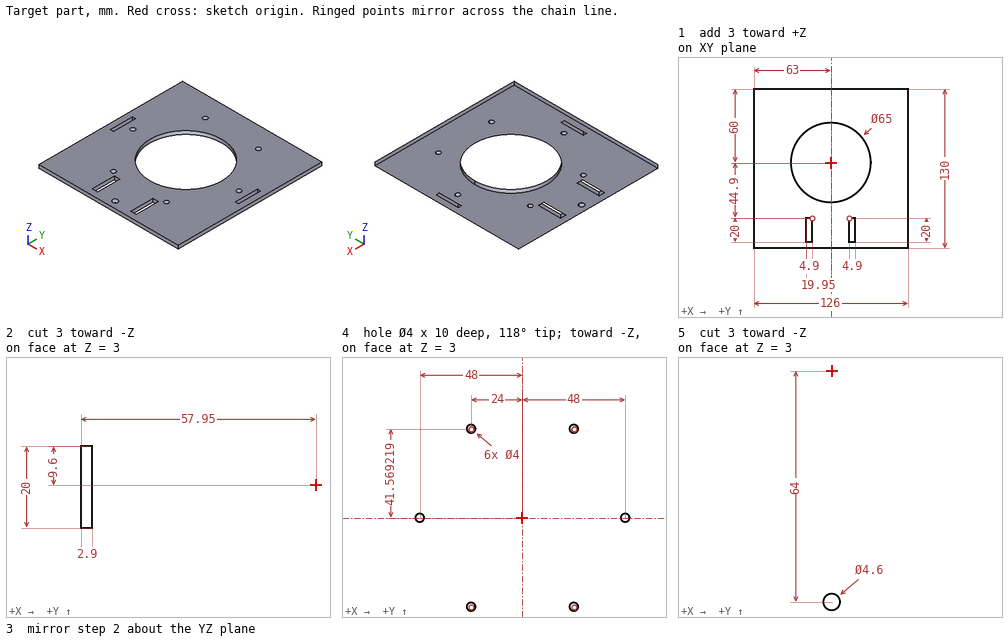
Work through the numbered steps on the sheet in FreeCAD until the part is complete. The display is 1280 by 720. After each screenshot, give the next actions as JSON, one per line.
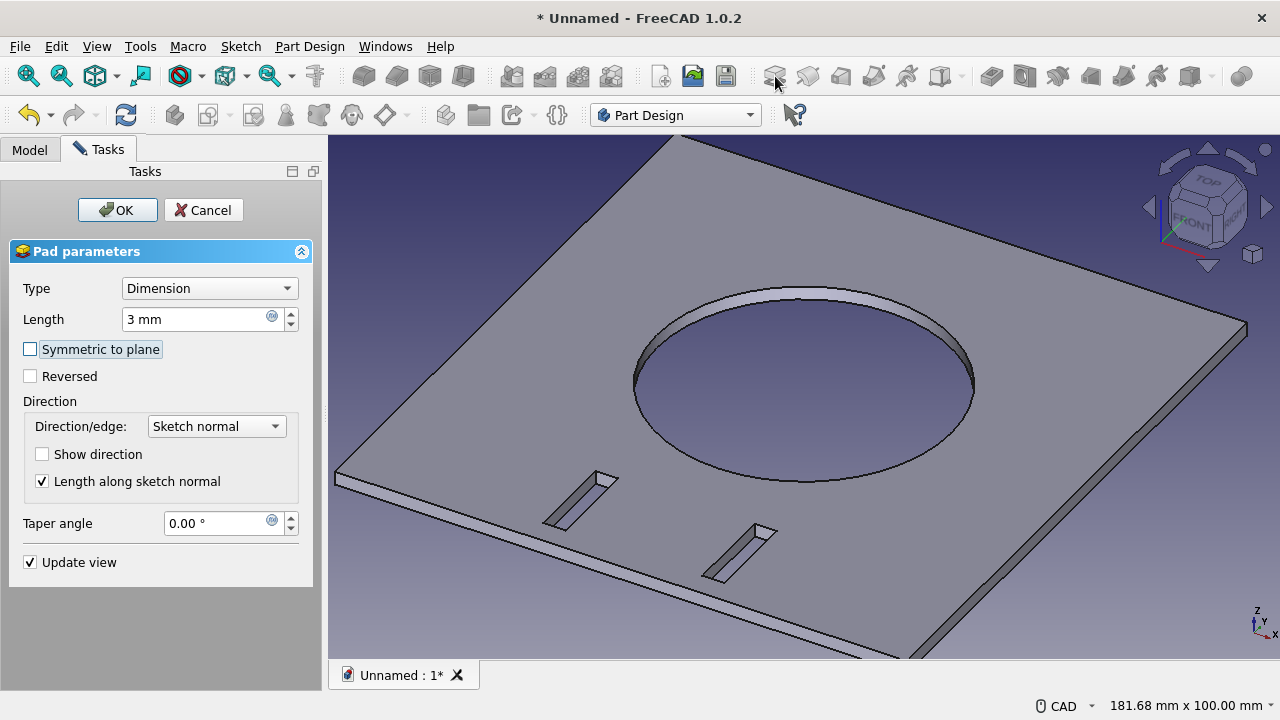
{"action": "left_click", "coordinate": [118, 210]}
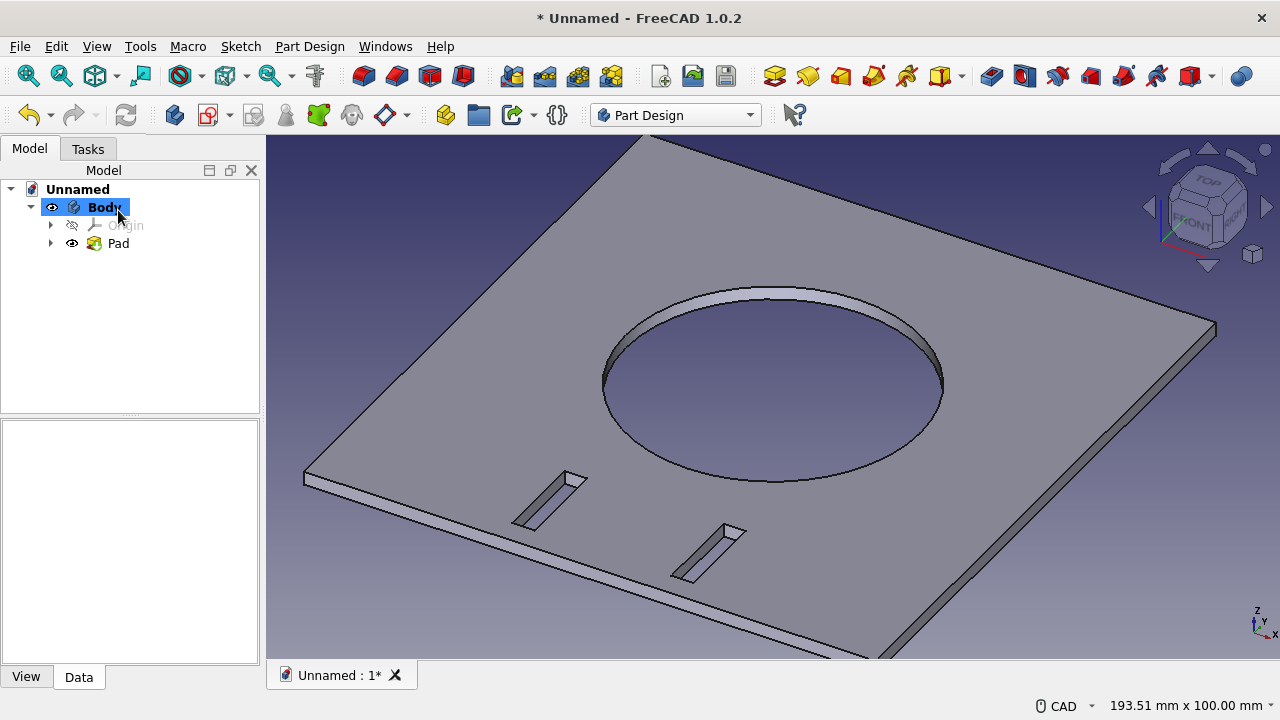
{"action": "left_click", "coordinate": [29, 76]}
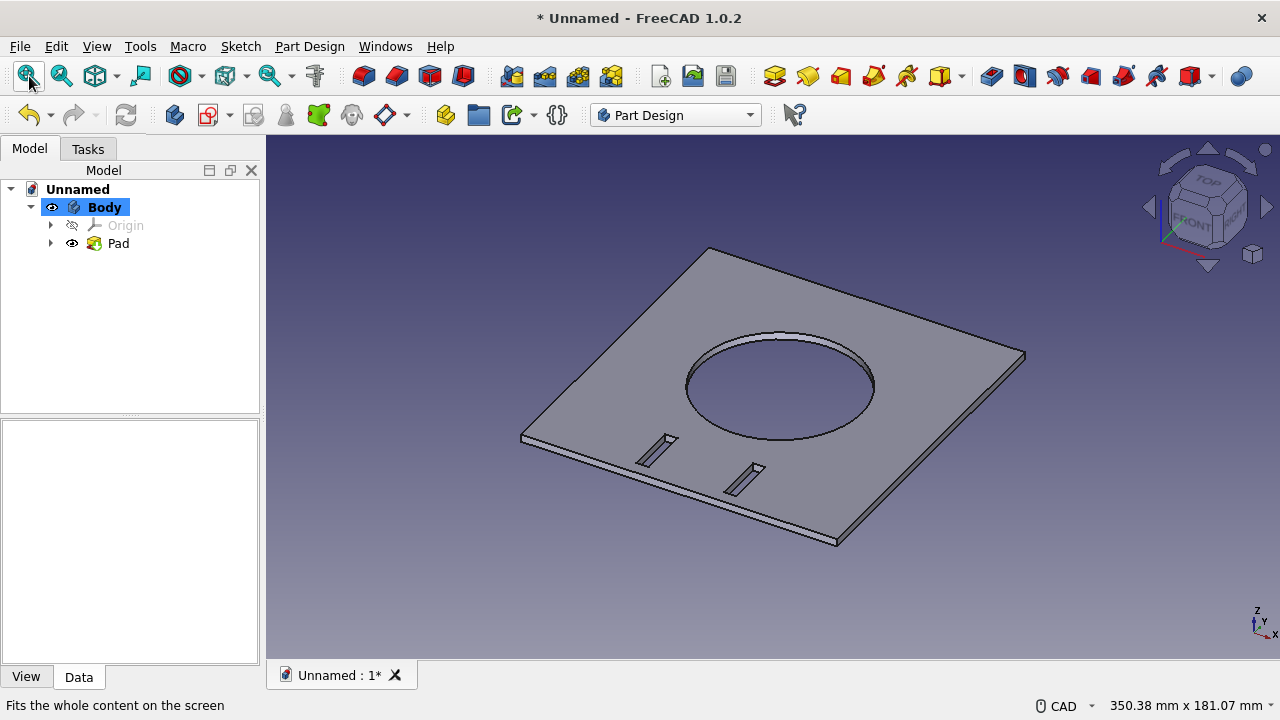
{"action": "left_click", "coordinate": [809, 476]}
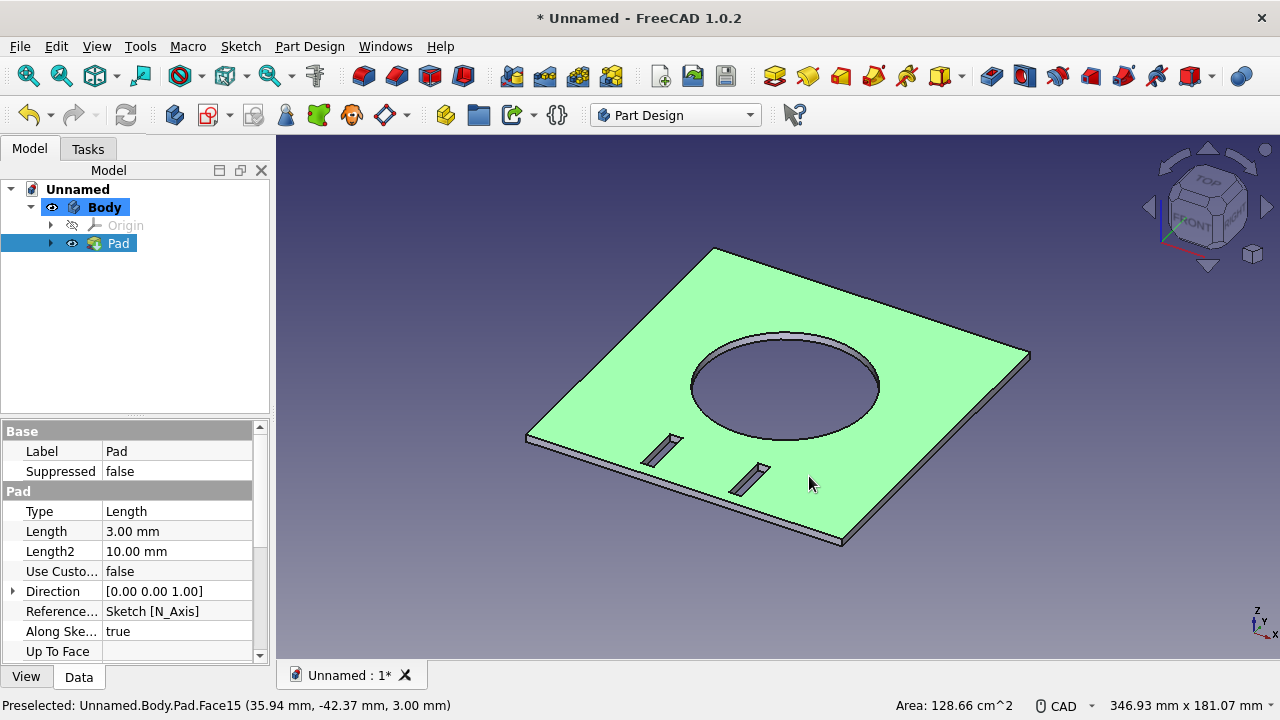
{"action": "left_click", "coordinate": [208, 116]}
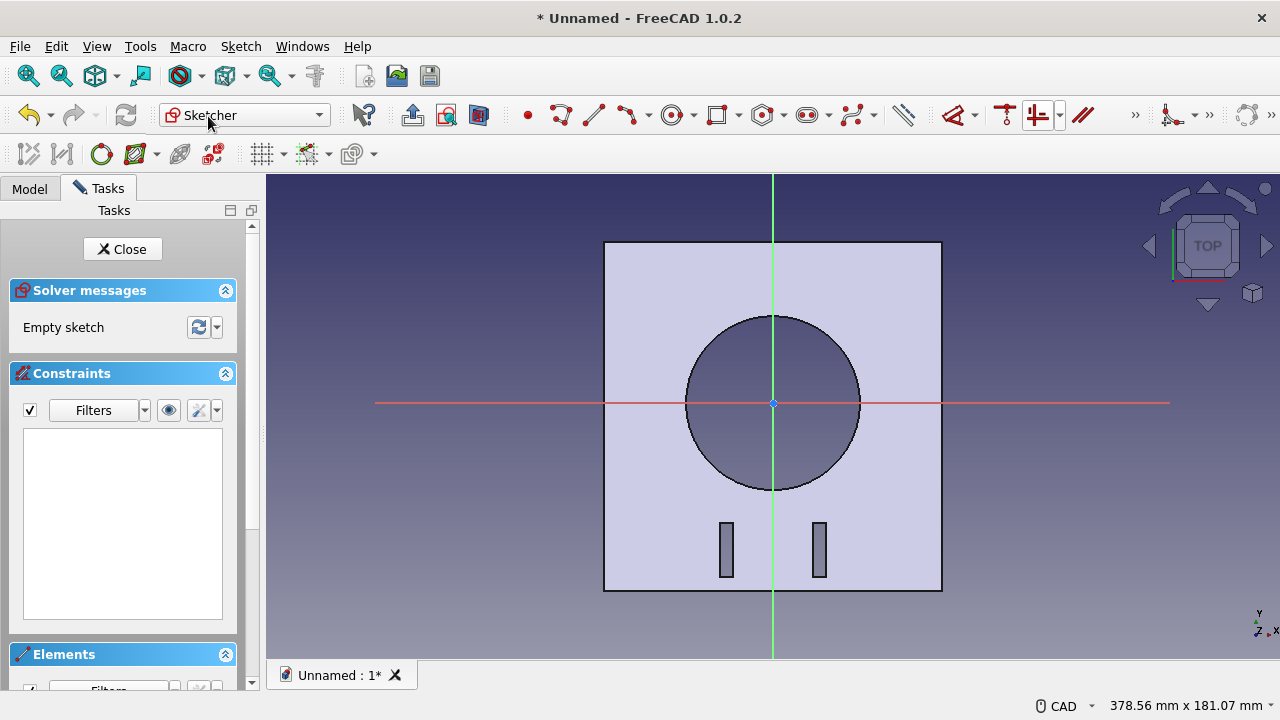
{"action": "scroll", "coordinate": [605, 402], "scroll_direction": "up", "scroll_amount": 9}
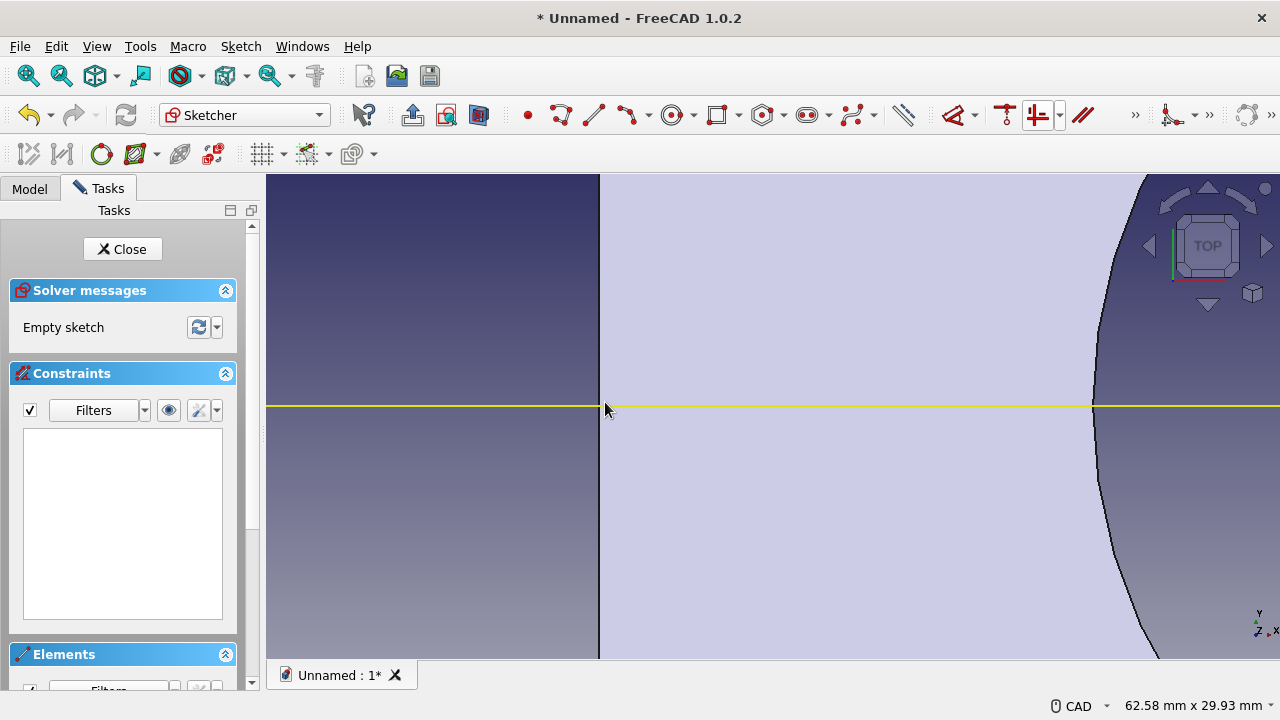
{"action": "left_click", "coordinate": [716, 116]}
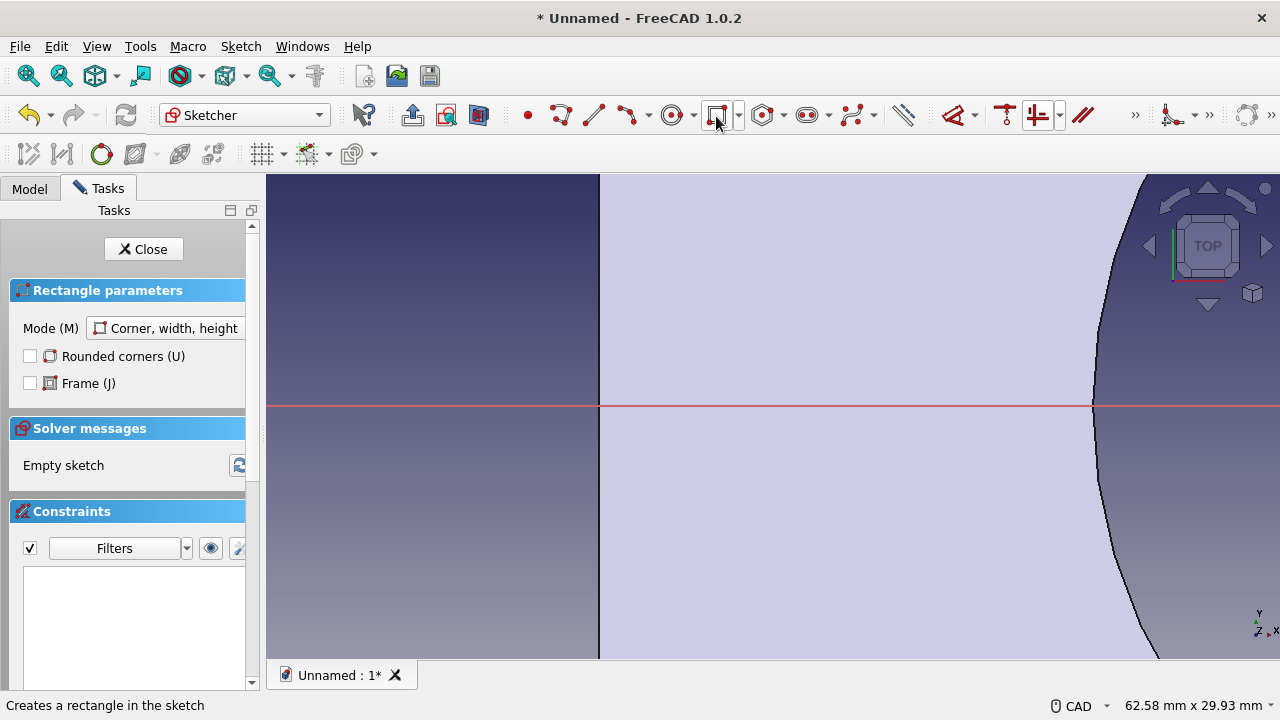
{"action": "left_click", "coordinate": [681, 251]}
{"action": "mouse_move", "coordinate": [728, 575]}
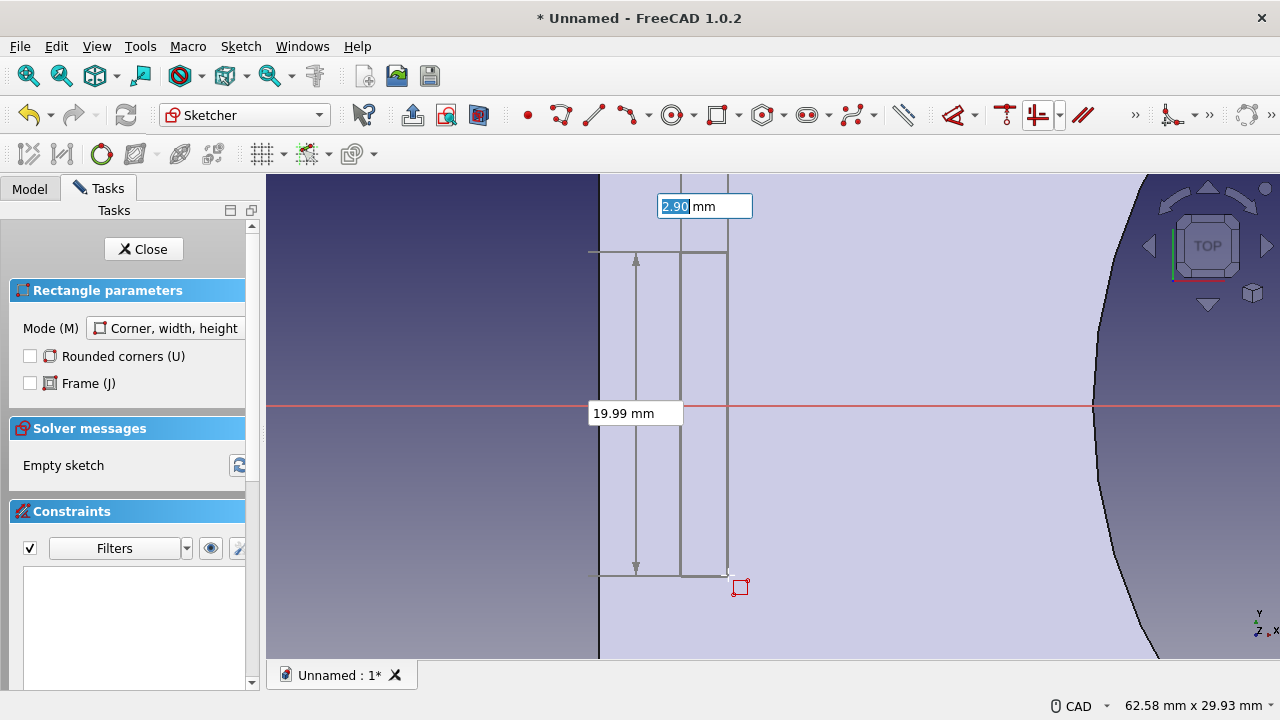
{"action": "type", "text": "2.9"}
{"action": "key", "text": "Tab"}
{"action": "type", "text": "20"}
{"action": "key", "text": "Return"}
{"action": "key", "text": "Escape"}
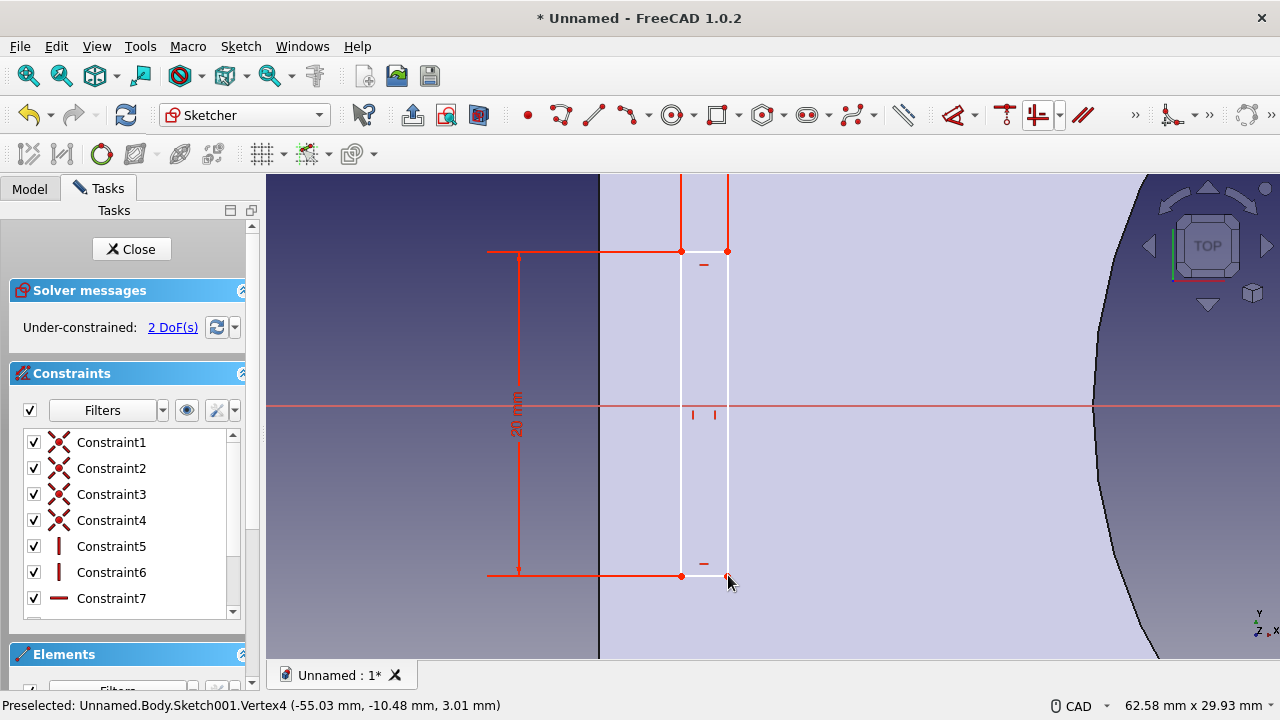
{"action": "left_click", "coordinate": [952, 116]}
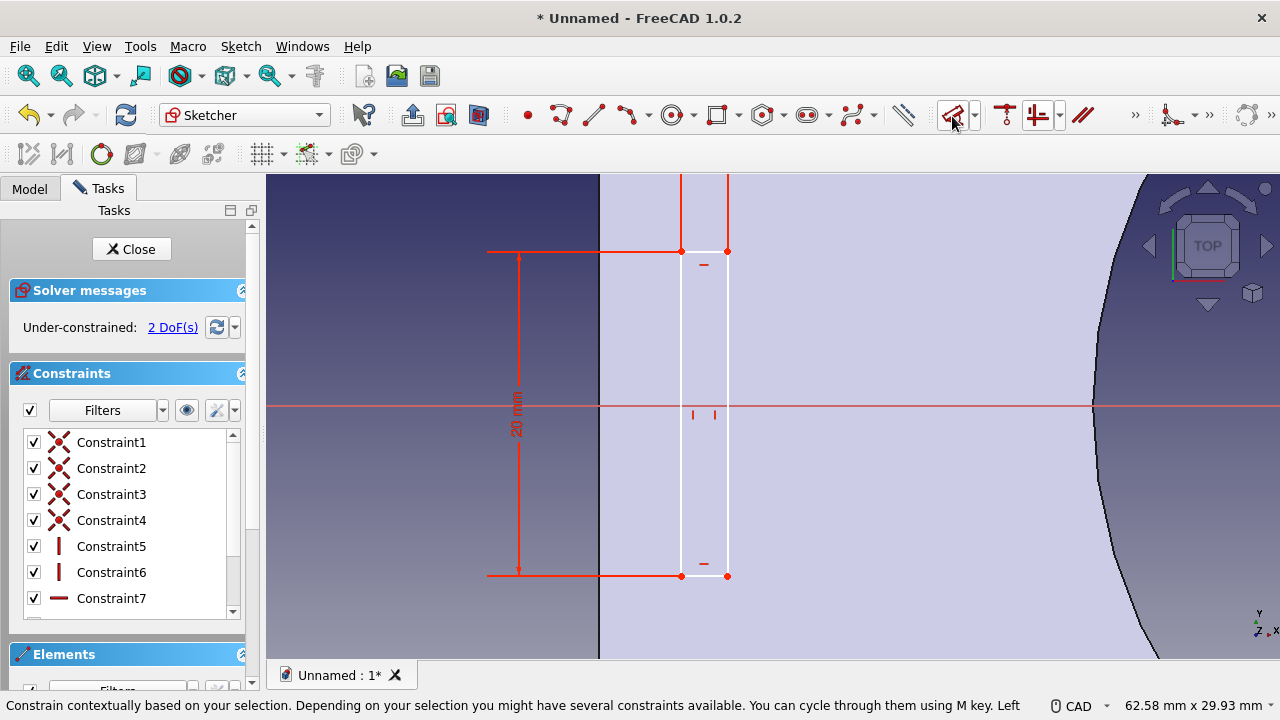
{"action": "left_click", "coordinate": [681, 252]}
{"action": "left_click", "coordinate": [647, 329]}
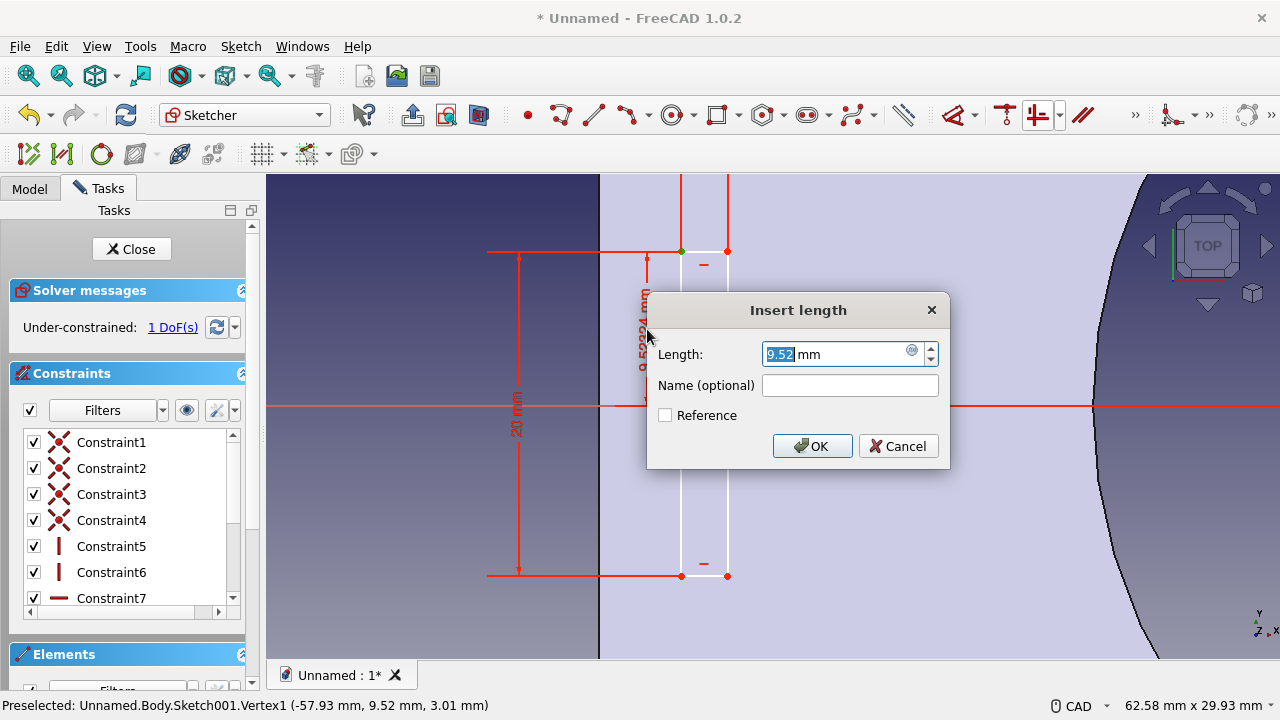
{"action": "type", "text": "9.6"}
{"action": "key", "text": "Return"}